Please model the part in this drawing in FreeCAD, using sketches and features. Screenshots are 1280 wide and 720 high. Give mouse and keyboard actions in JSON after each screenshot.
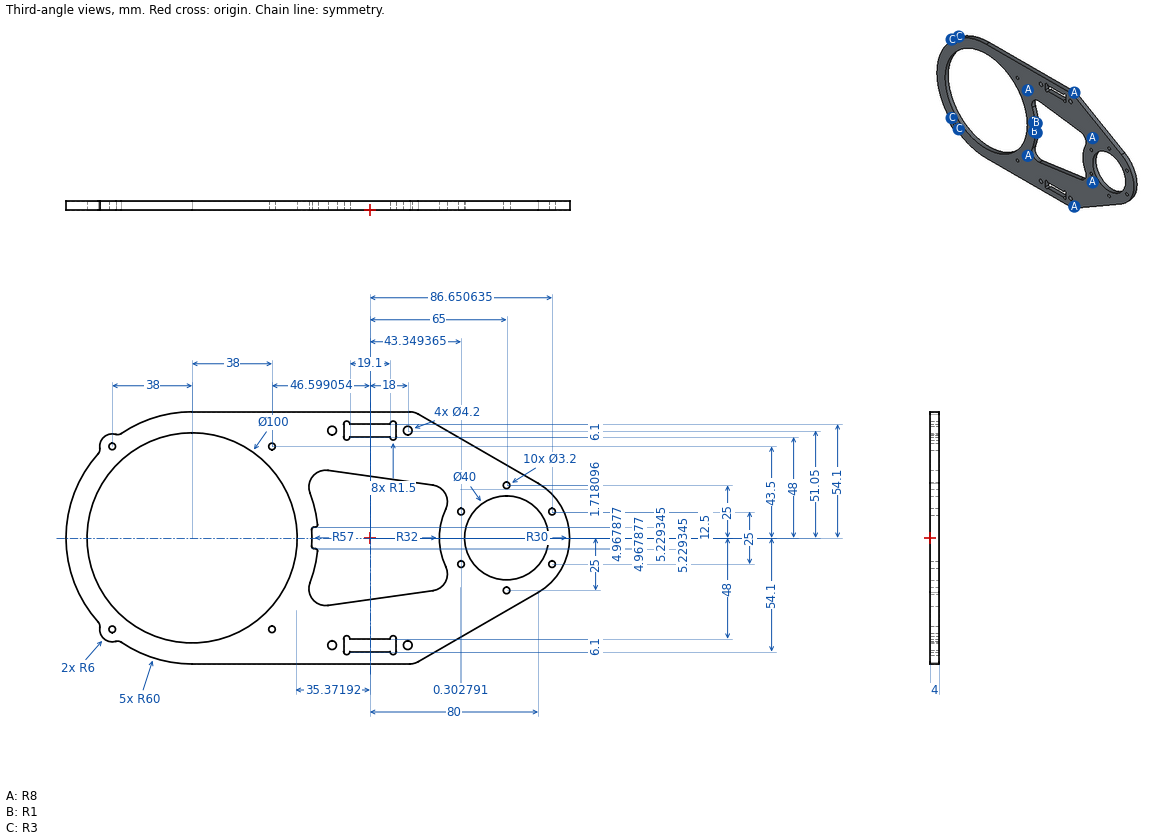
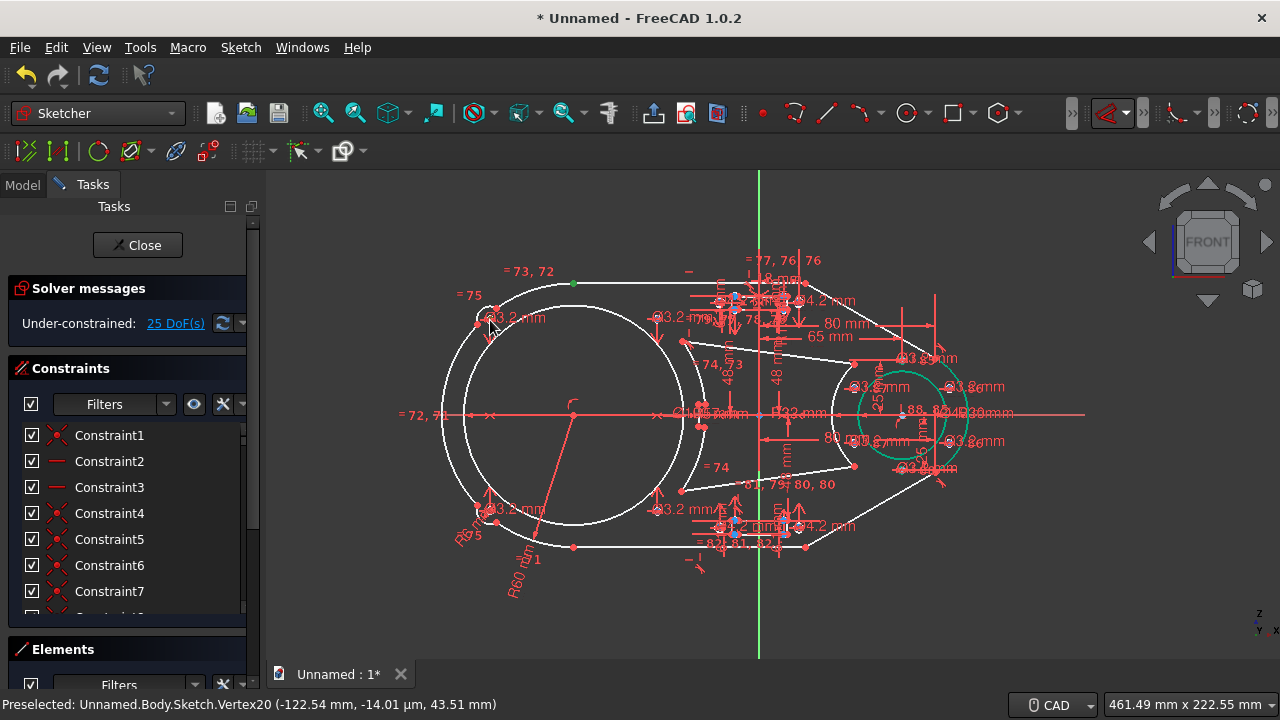
{"action": "left_click", "coordinate": [1128, 114]}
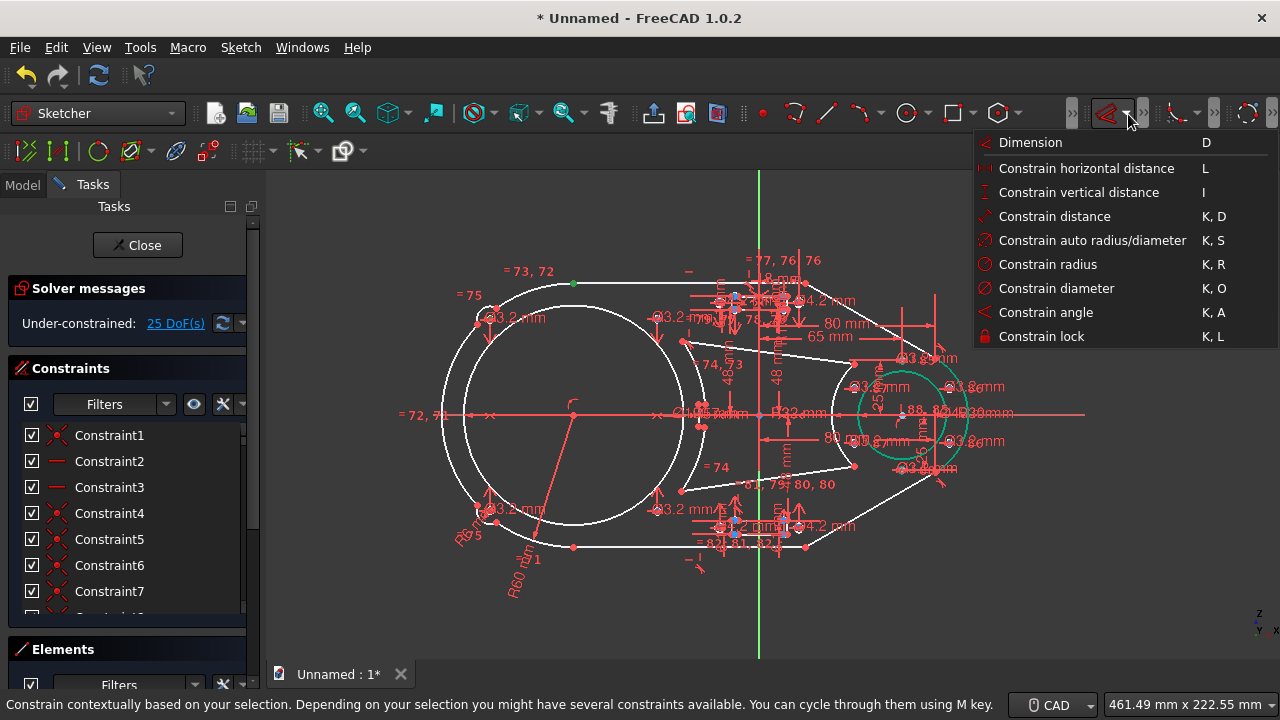
{"action": "left_click", "coordinate": [1126, 168]}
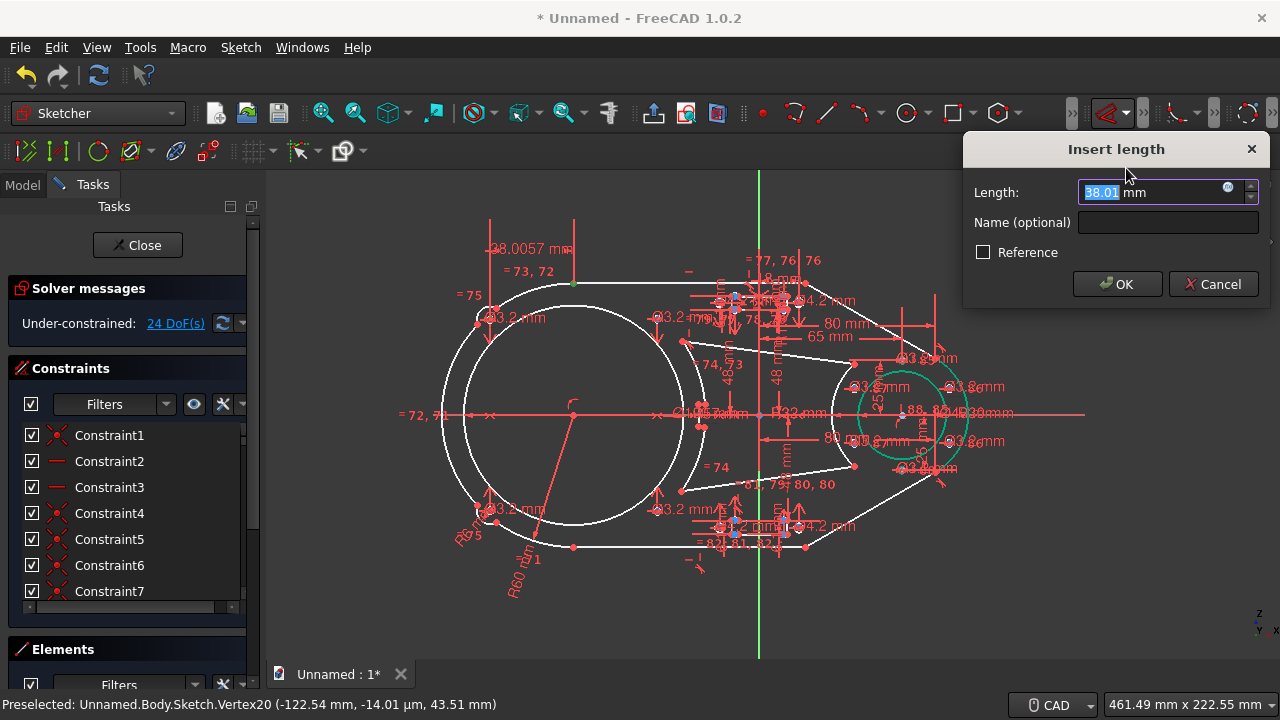
{"action": "type", "text": "38"}
{"action": "key", "text": "Return"}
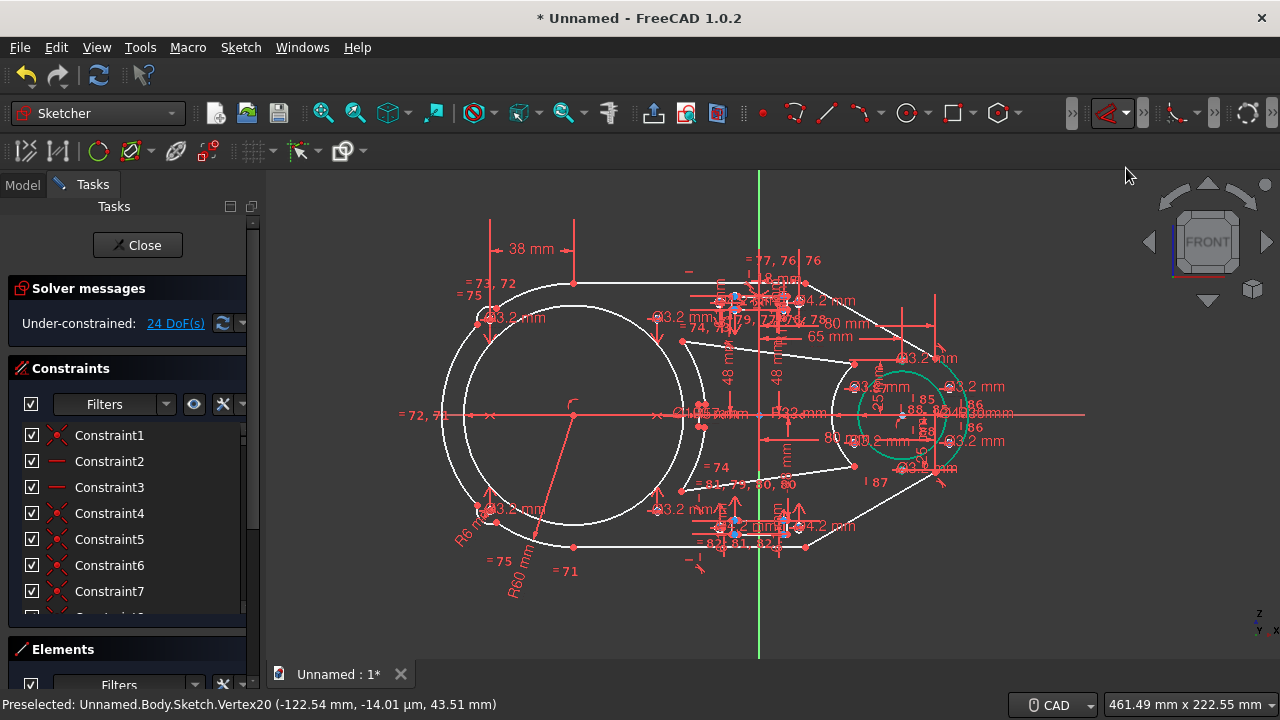
{"action": "left_click", "coordinate": [950, 389]}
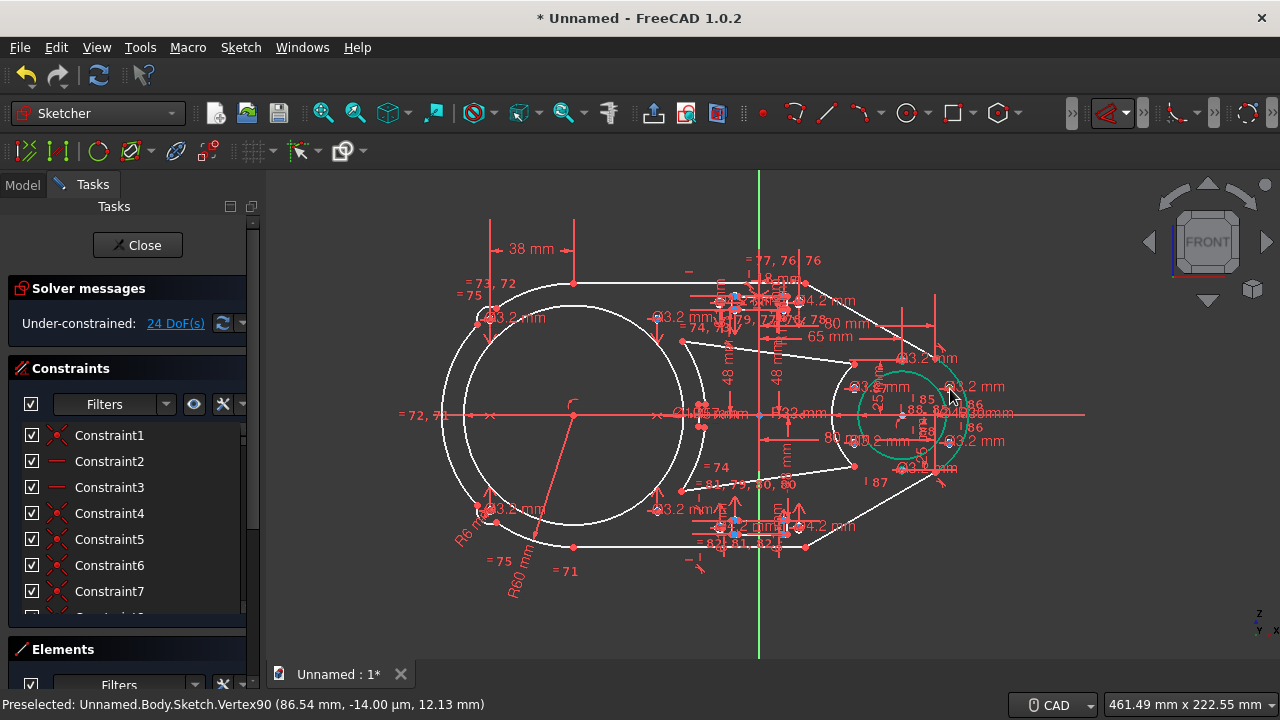
{"action": "left_click", "coordinate": [950, 443]}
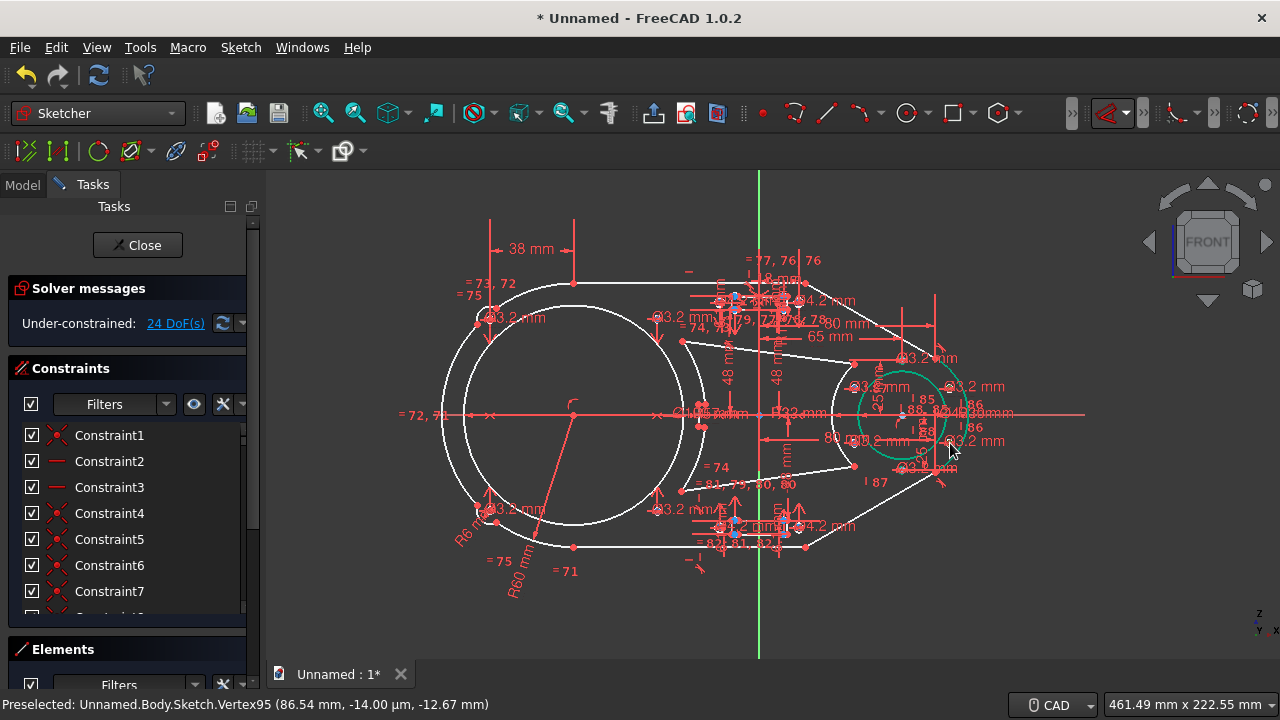
{"action": "left_click", "coordinate": [1128, 114]}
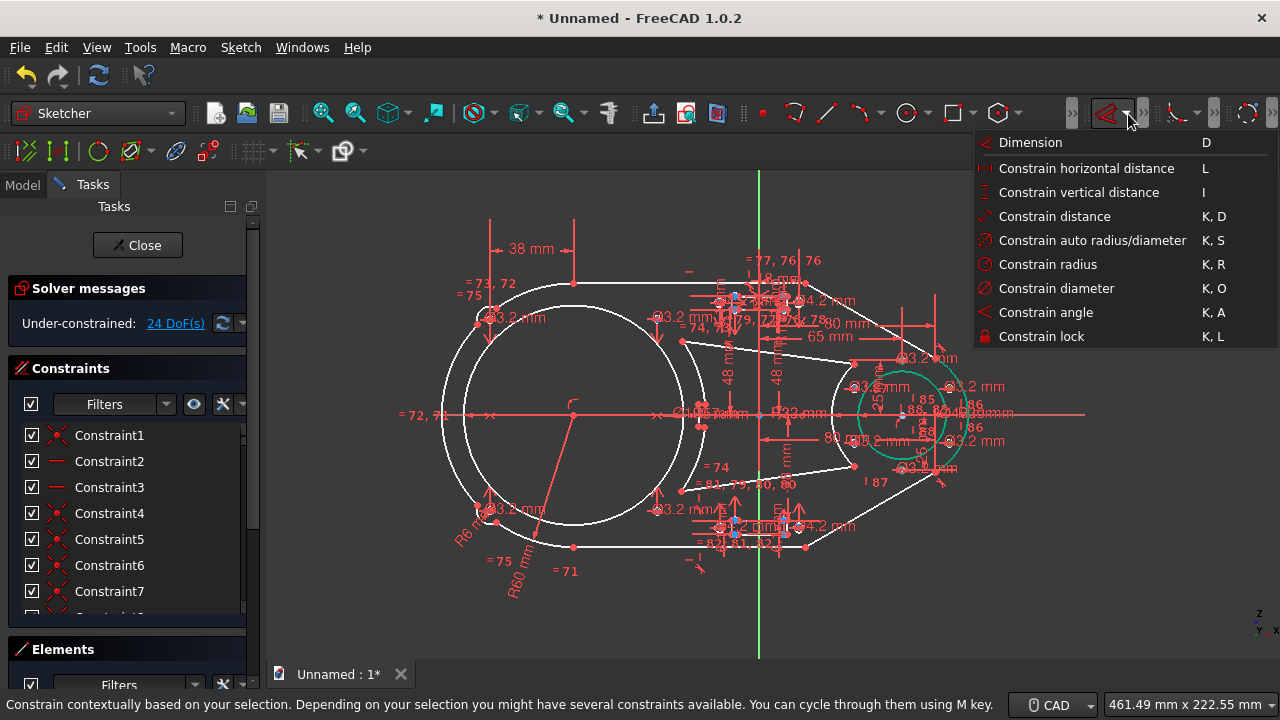
{"action": "left_click", "coordinate": [1126, 192]}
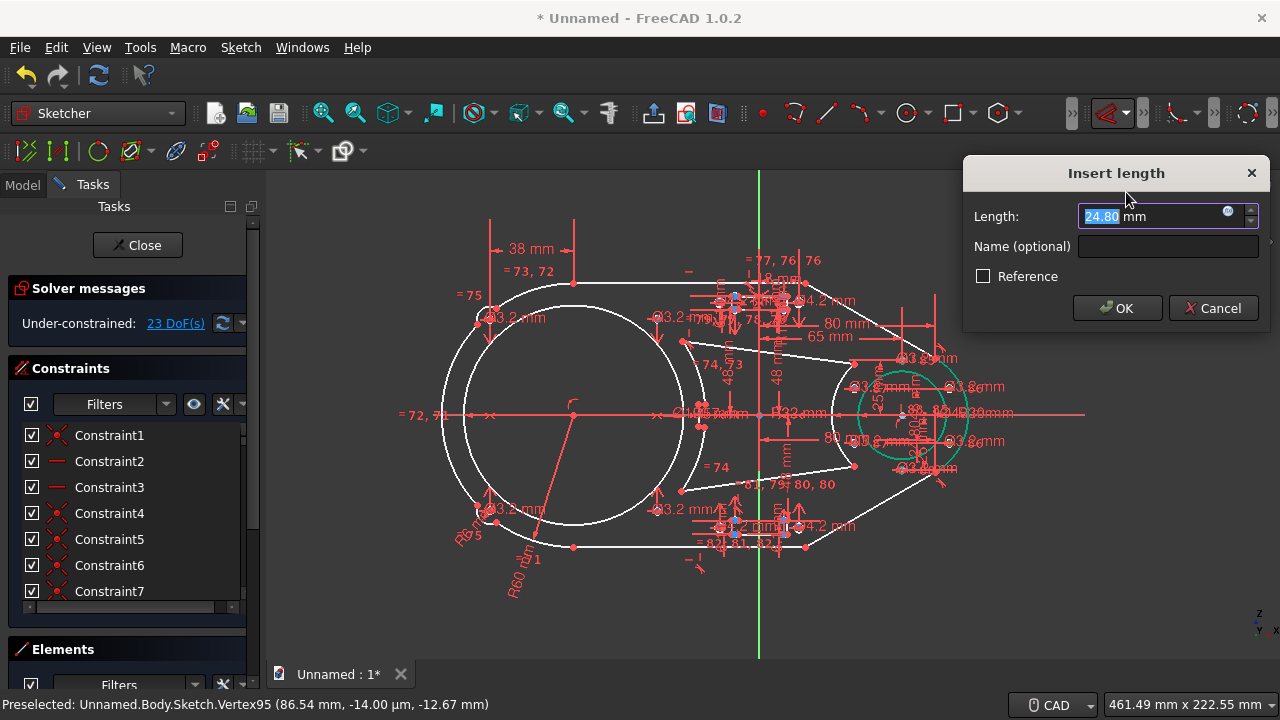
{"action": "type", "text": "25"}
{"action": "key", "text": "Return"}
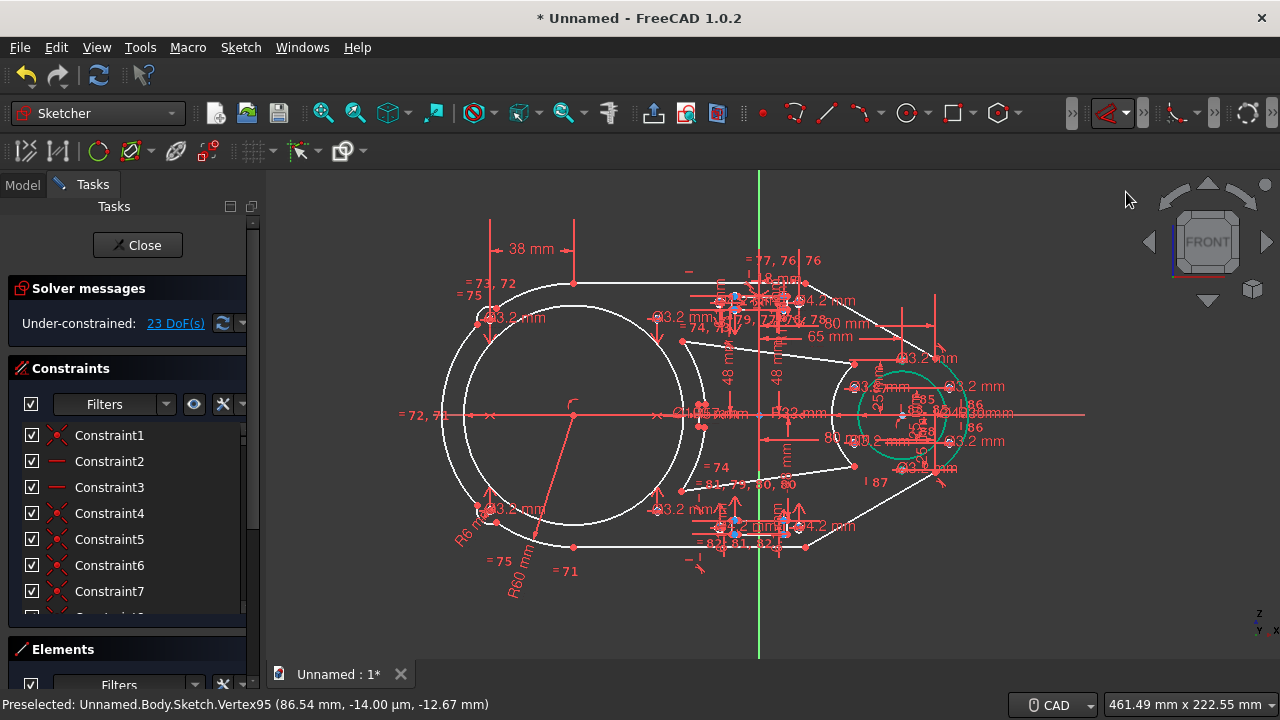
{"action": "left_click", "coordinate": [855, 389]}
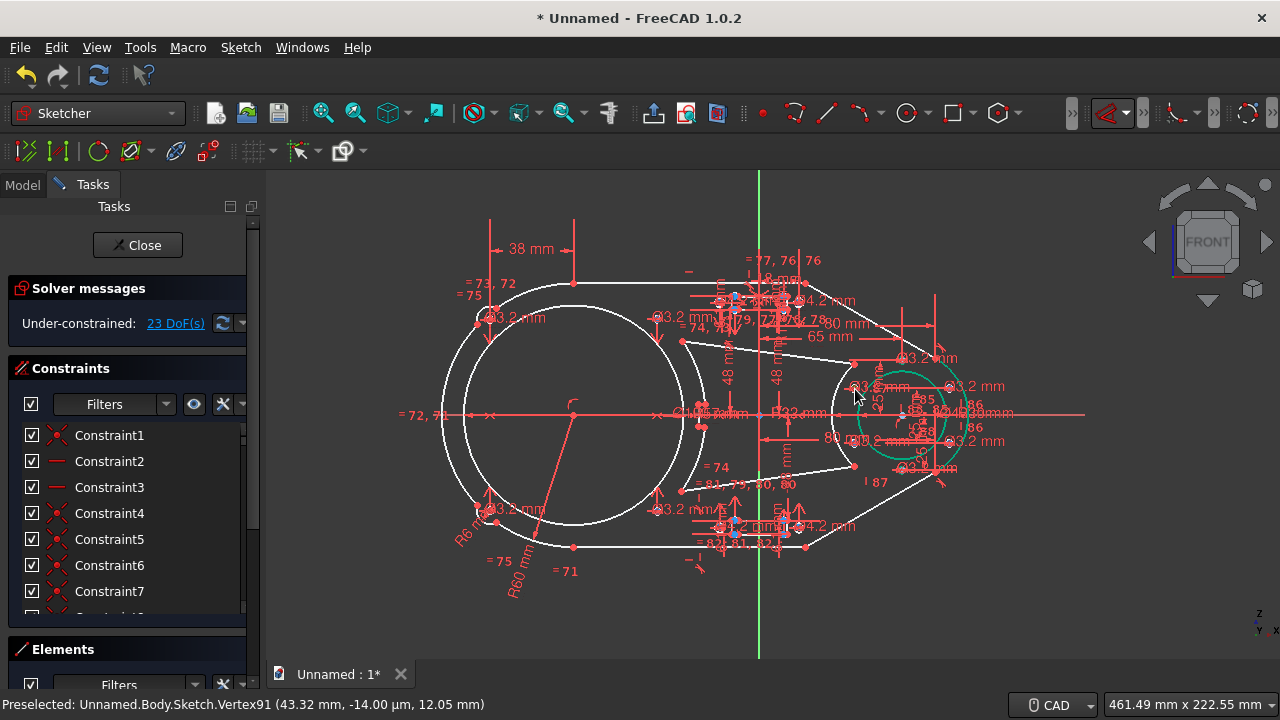
{"action": "left_click", "coordinate": [855, 443]}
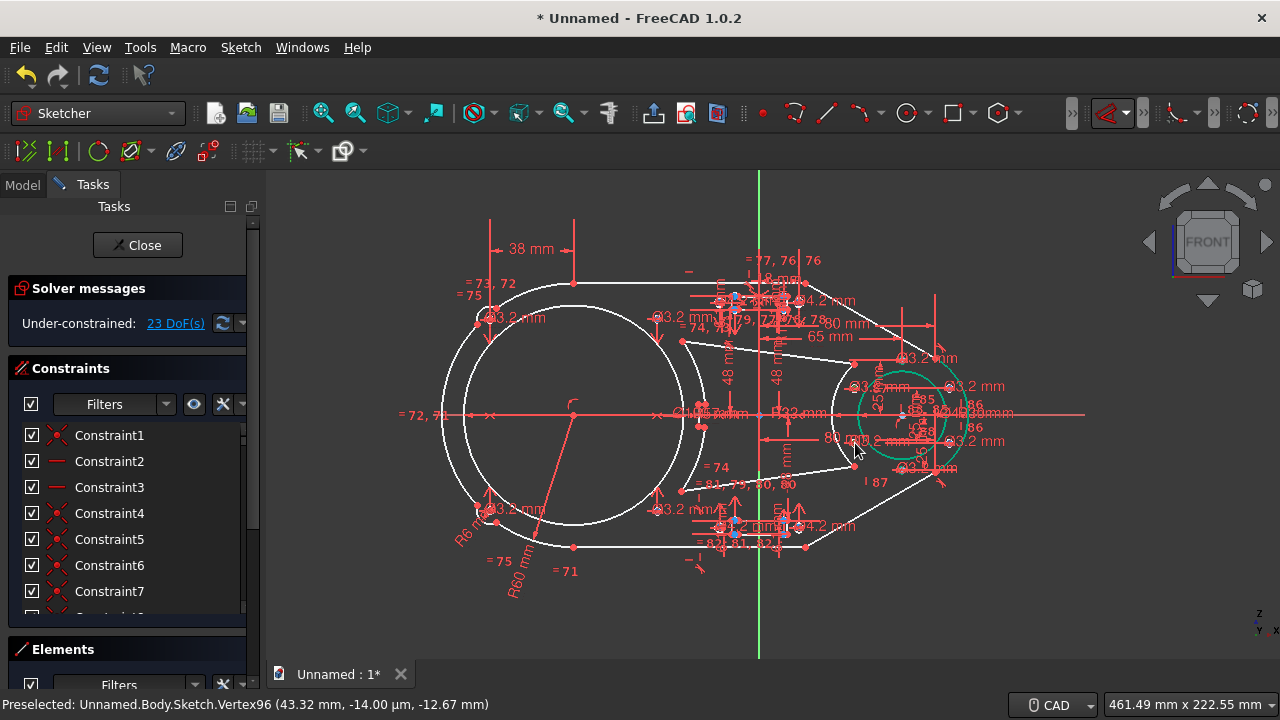
{"action": "left_click", "coordinate": [1128, 114]}